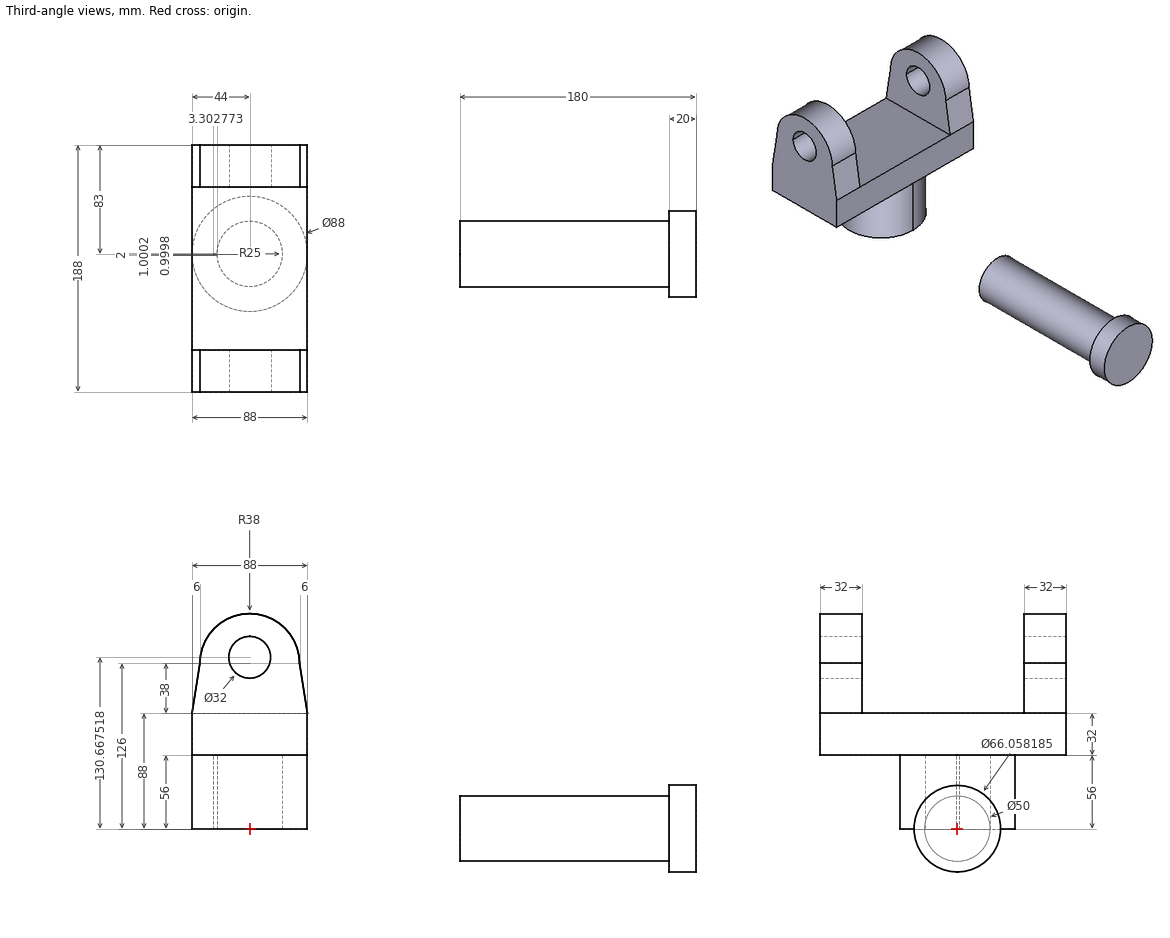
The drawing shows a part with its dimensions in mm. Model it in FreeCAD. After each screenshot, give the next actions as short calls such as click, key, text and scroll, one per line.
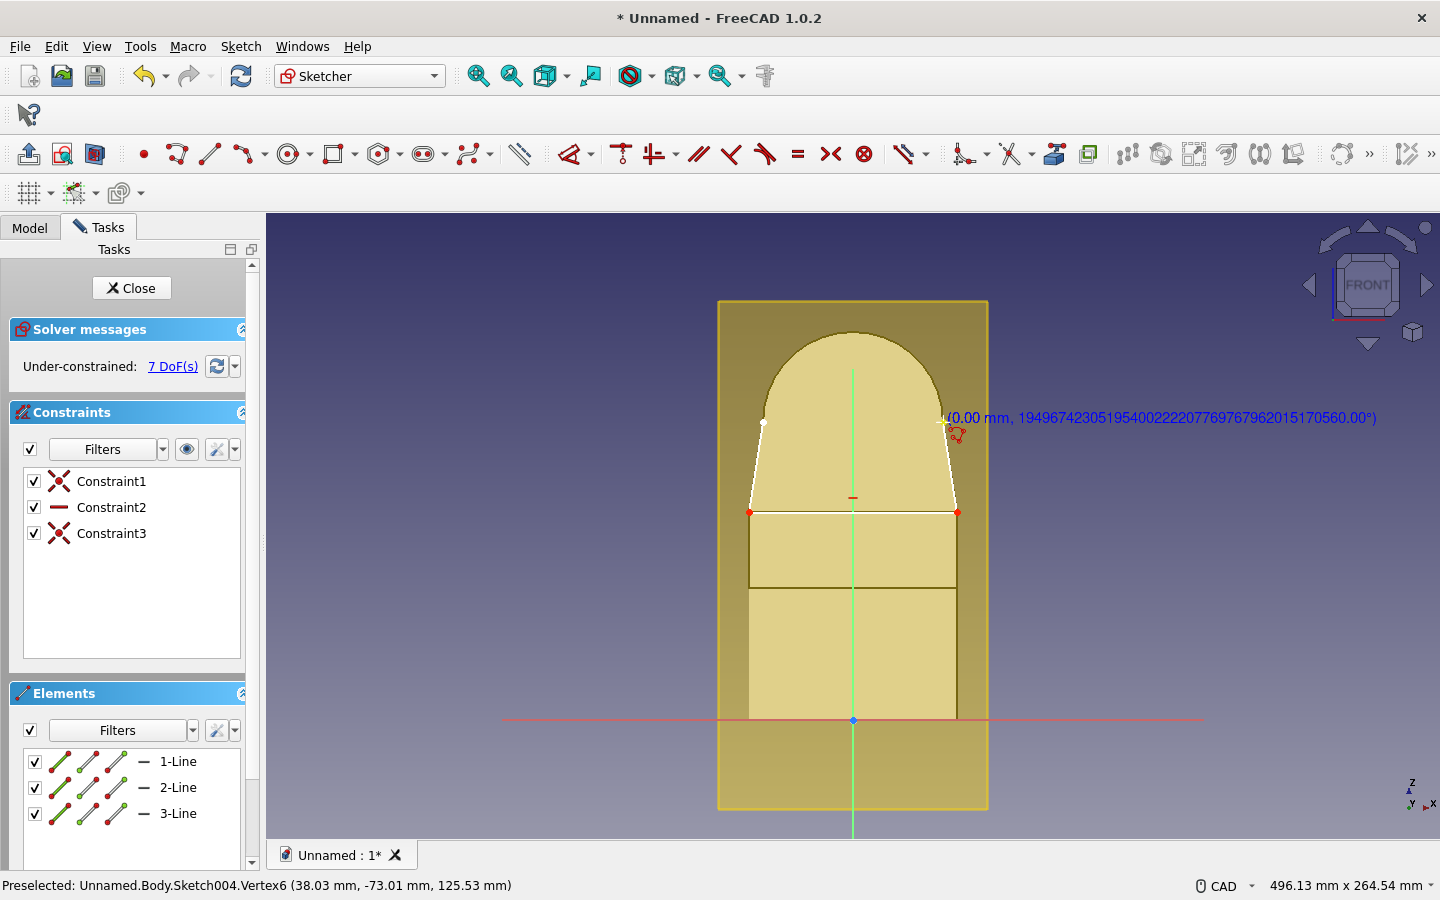
key(g)
key(3)
key(a)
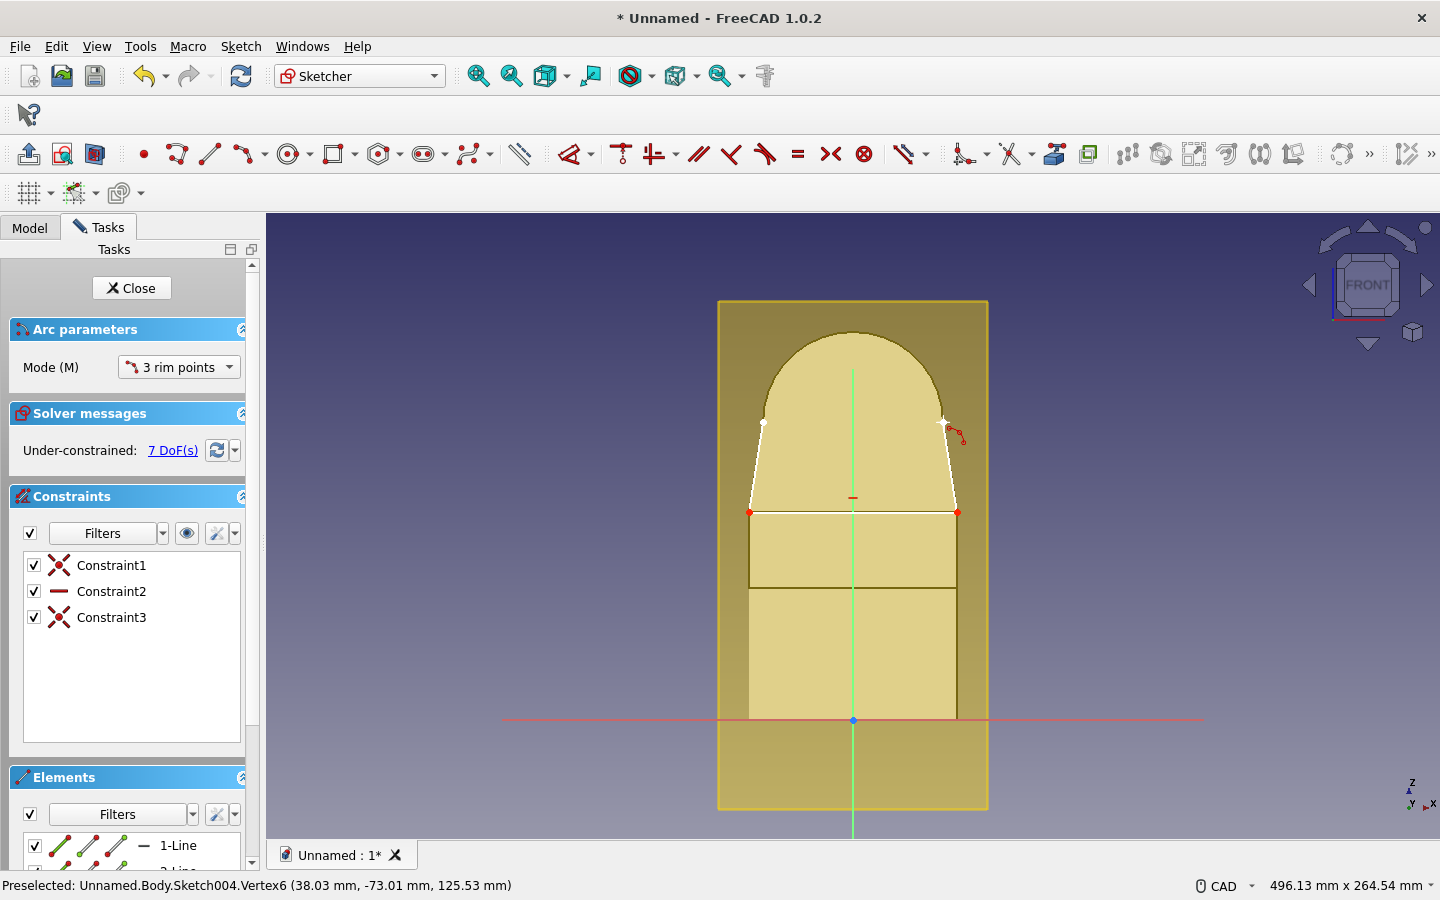
click(943, 423)
click(763, 423)
click(881, 336)
key(Escape)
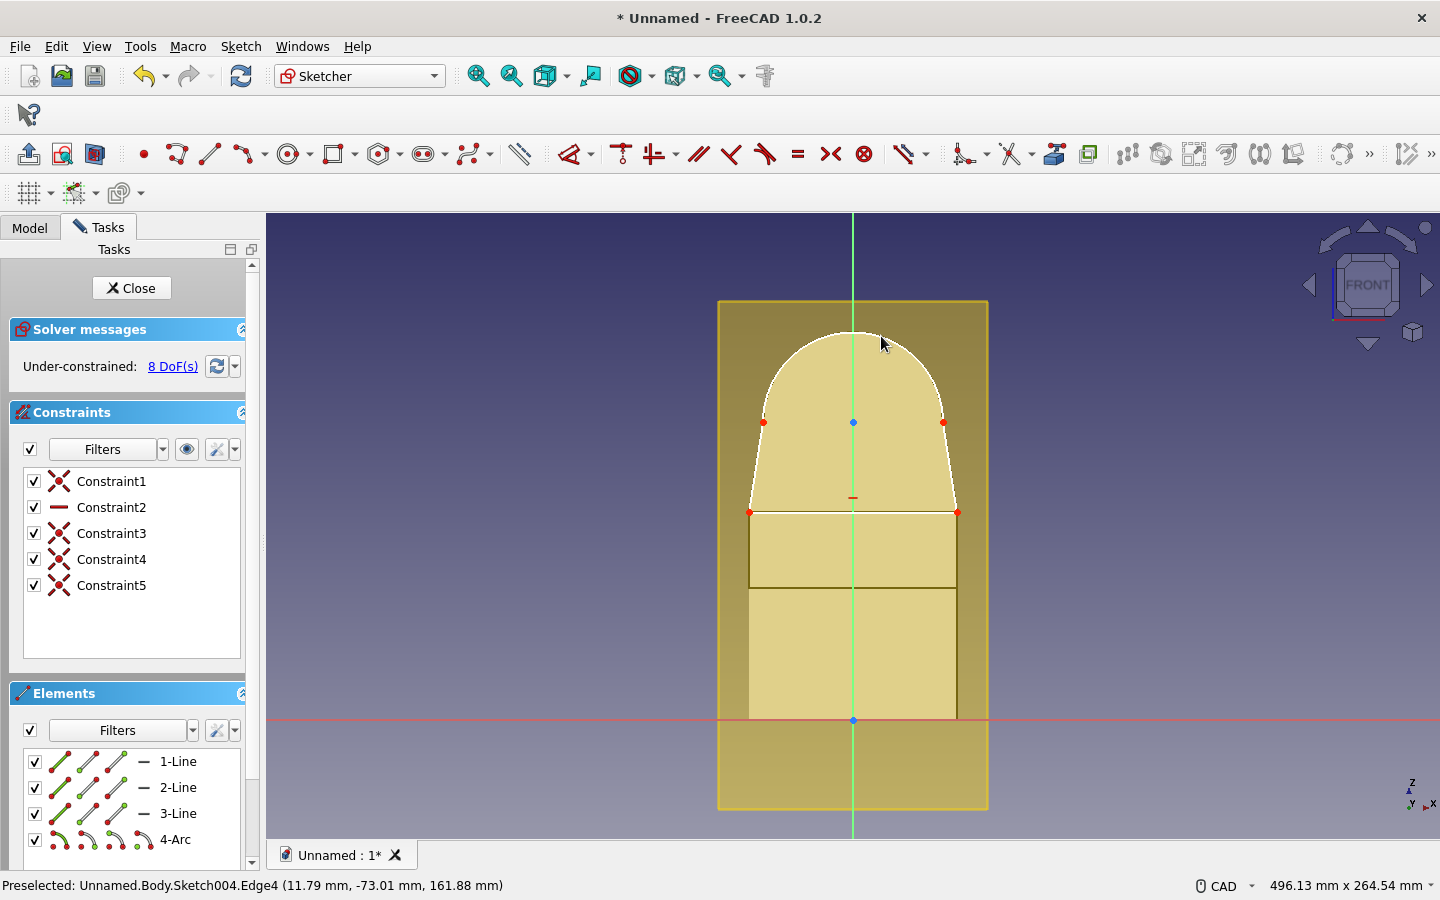
click(853, 423)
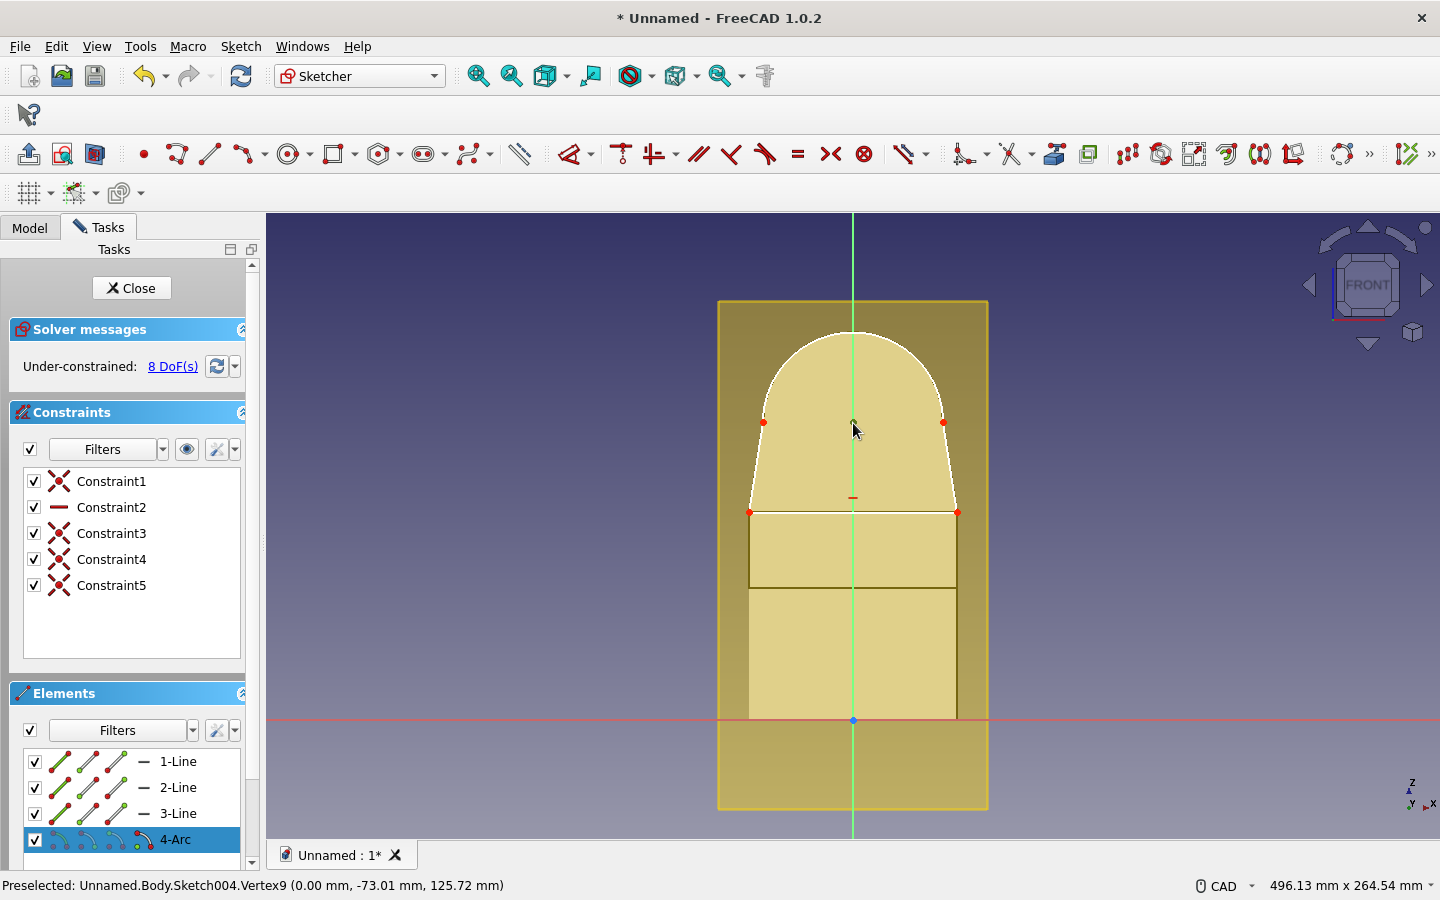
click(853, 770)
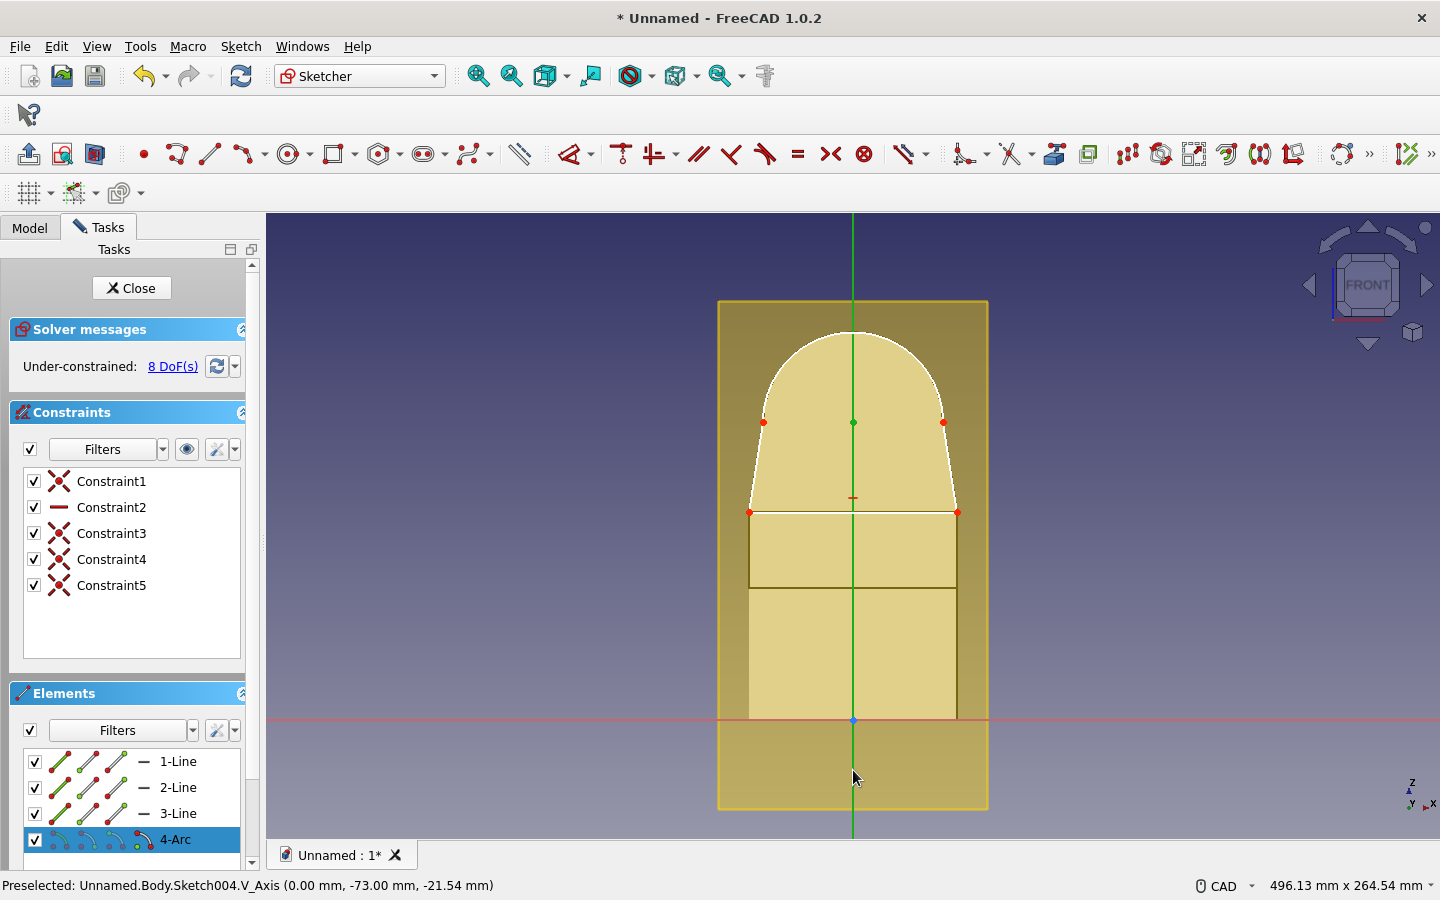
click(621, 154)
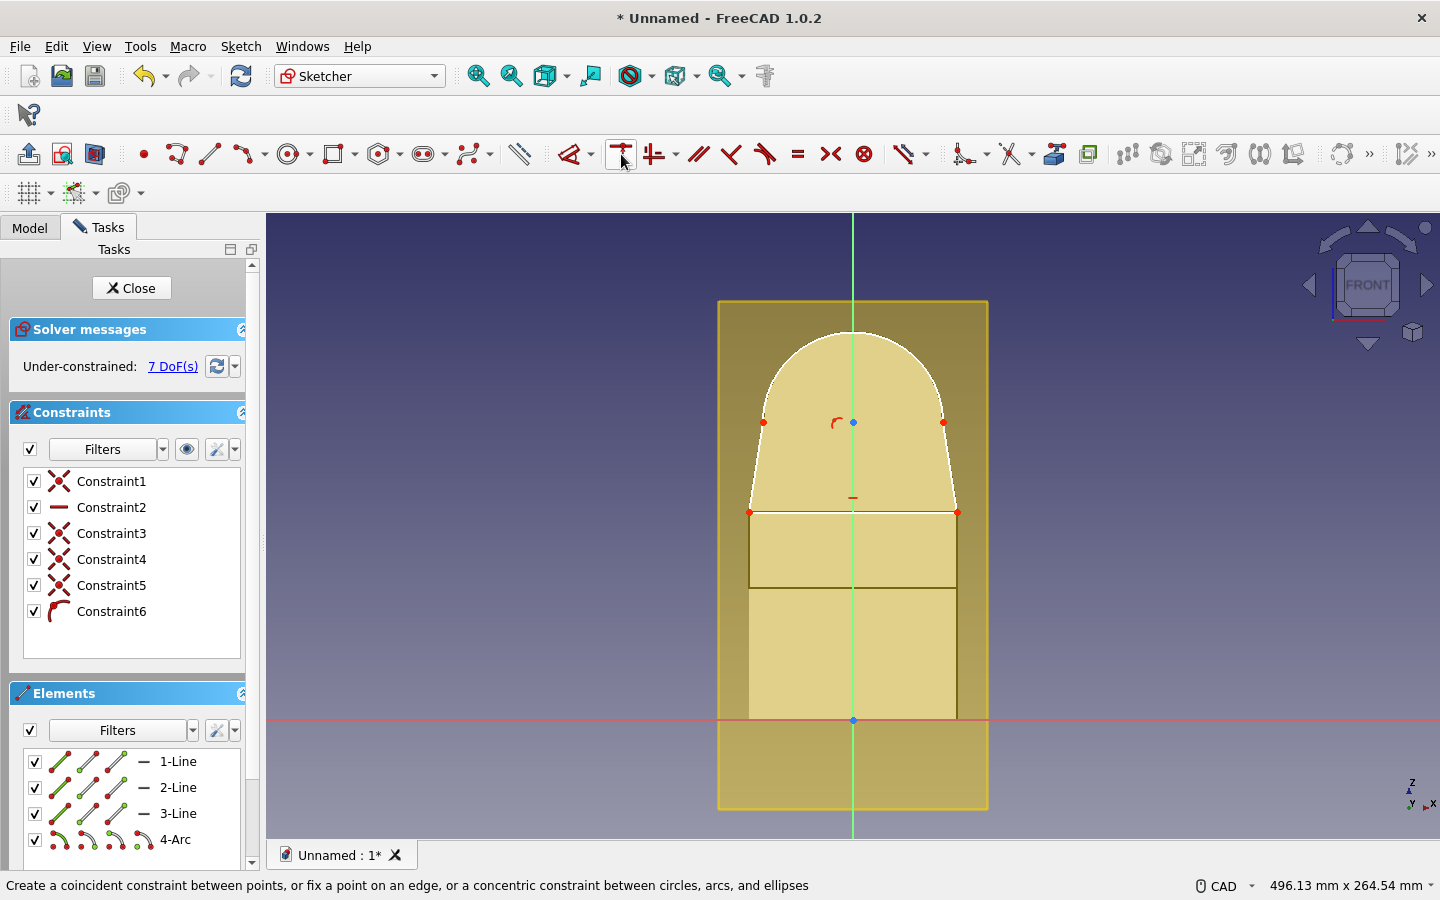
key(d)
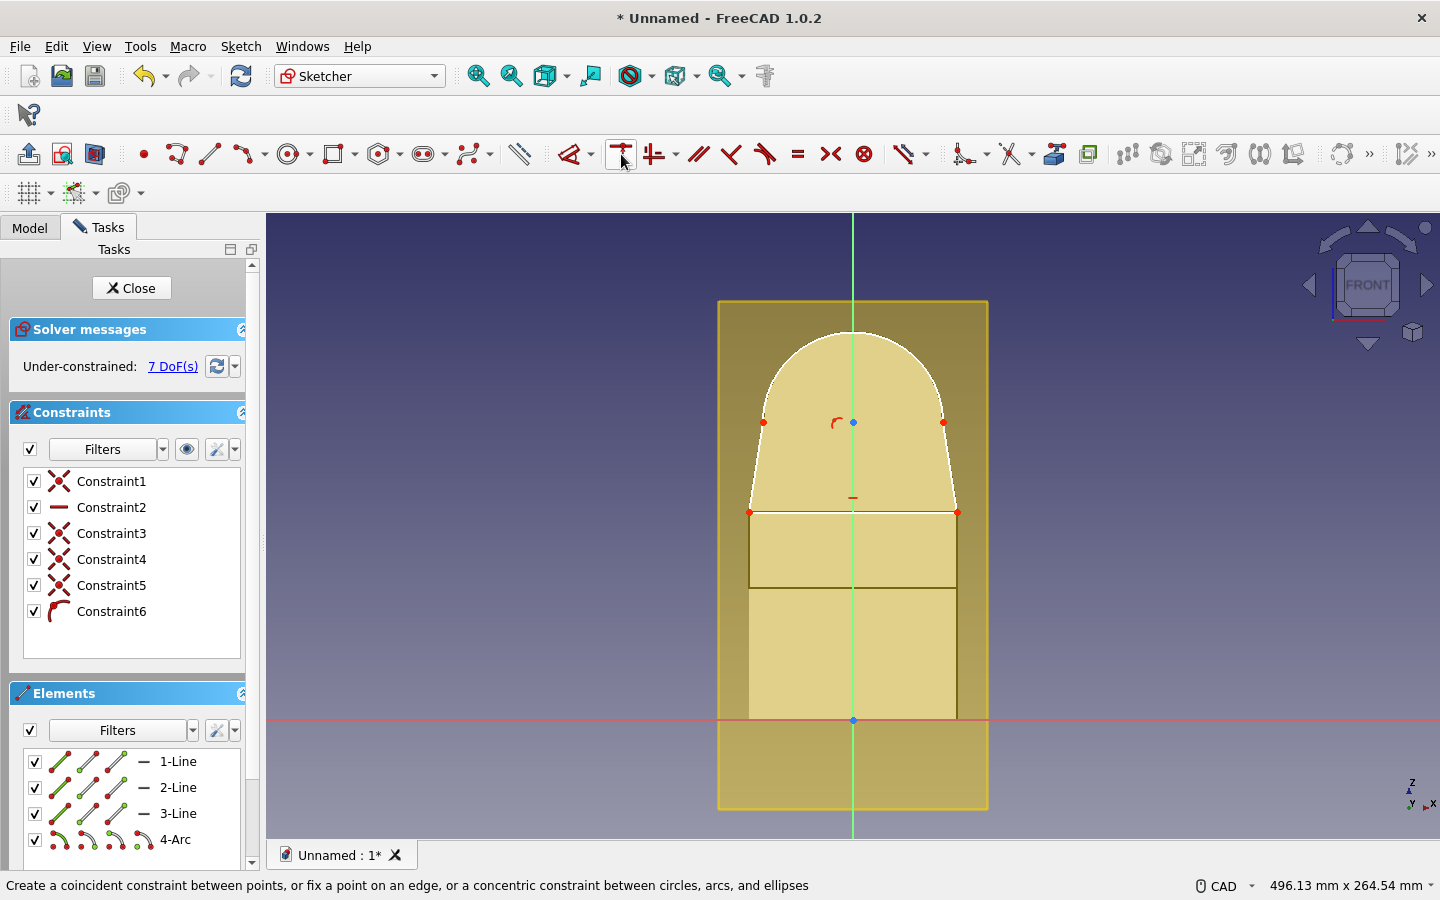
click(906, 350)
click(925, 324)